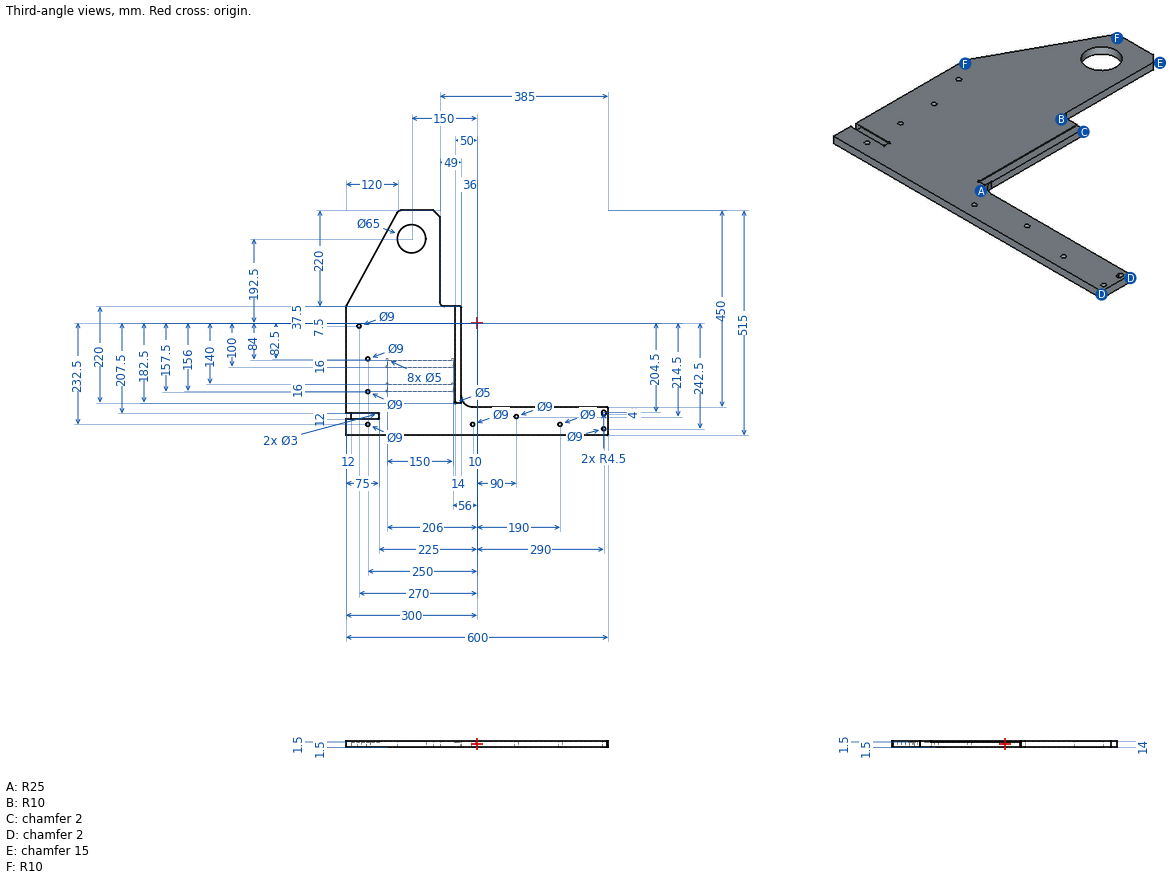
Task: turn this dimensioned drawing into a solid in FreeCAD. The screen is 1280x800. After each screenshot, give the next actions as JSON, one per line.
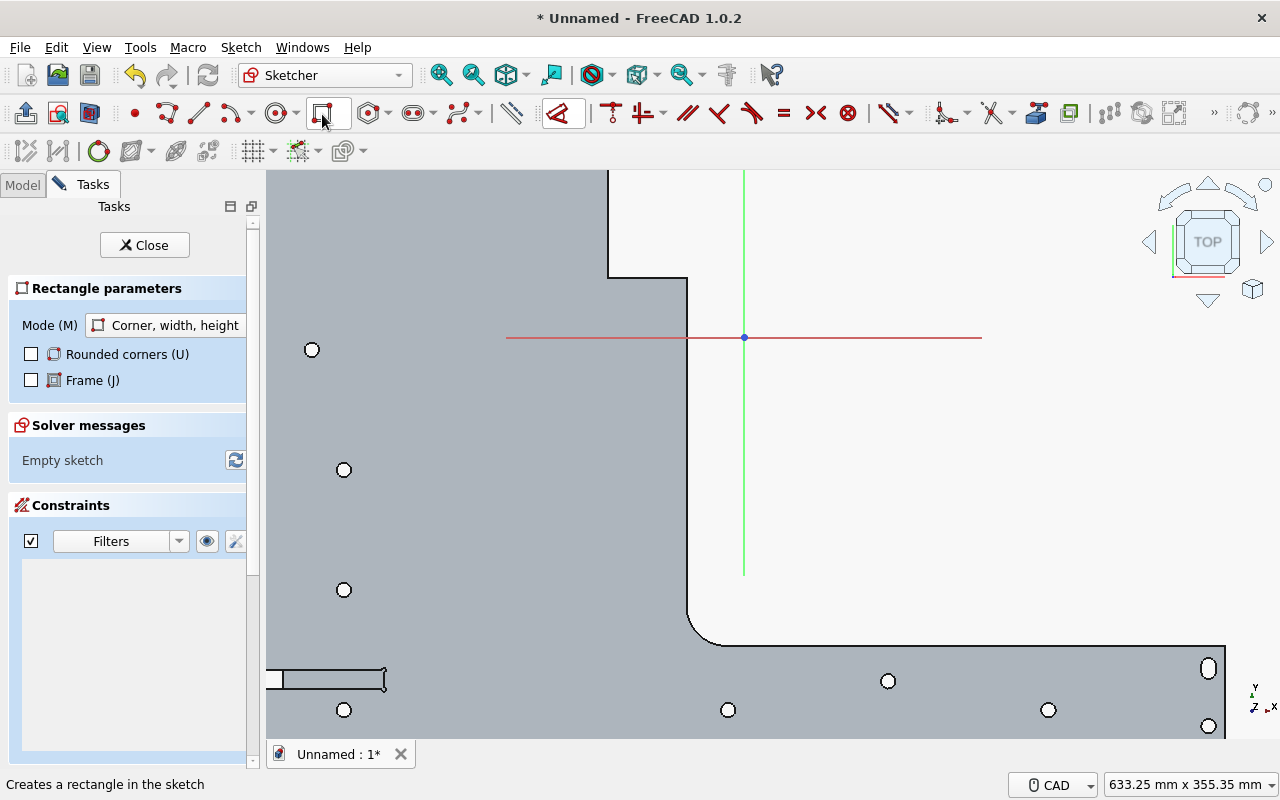
{"action": "left_click", "coordinate": [664, 278]}
{"action": "mouse_move", "coordinate": [687, 630]}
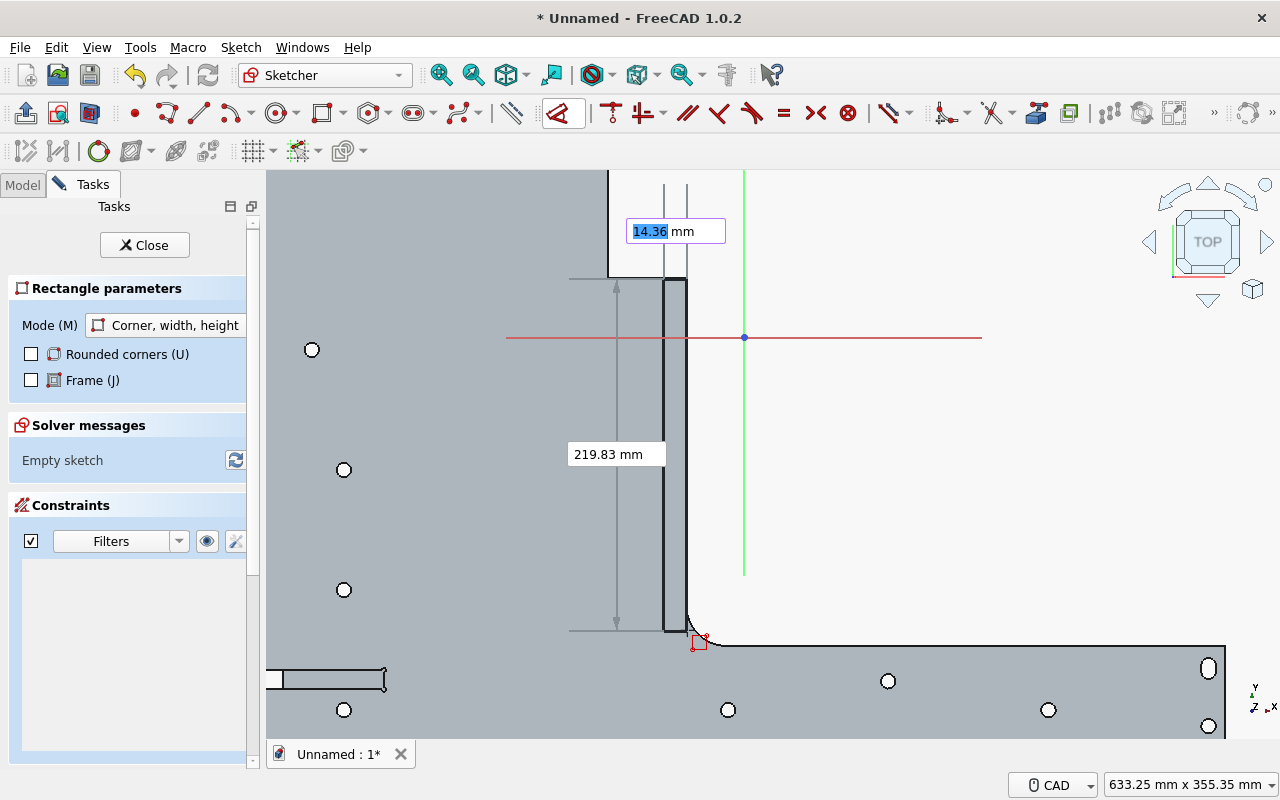
{"action": "type", "text": "14"}
{"action": "key", "text": "Tab"}
{"action": "type", "text": "220"}
{"action": "key", "text": "Return"}
{"action": "key", "text": "Escape"}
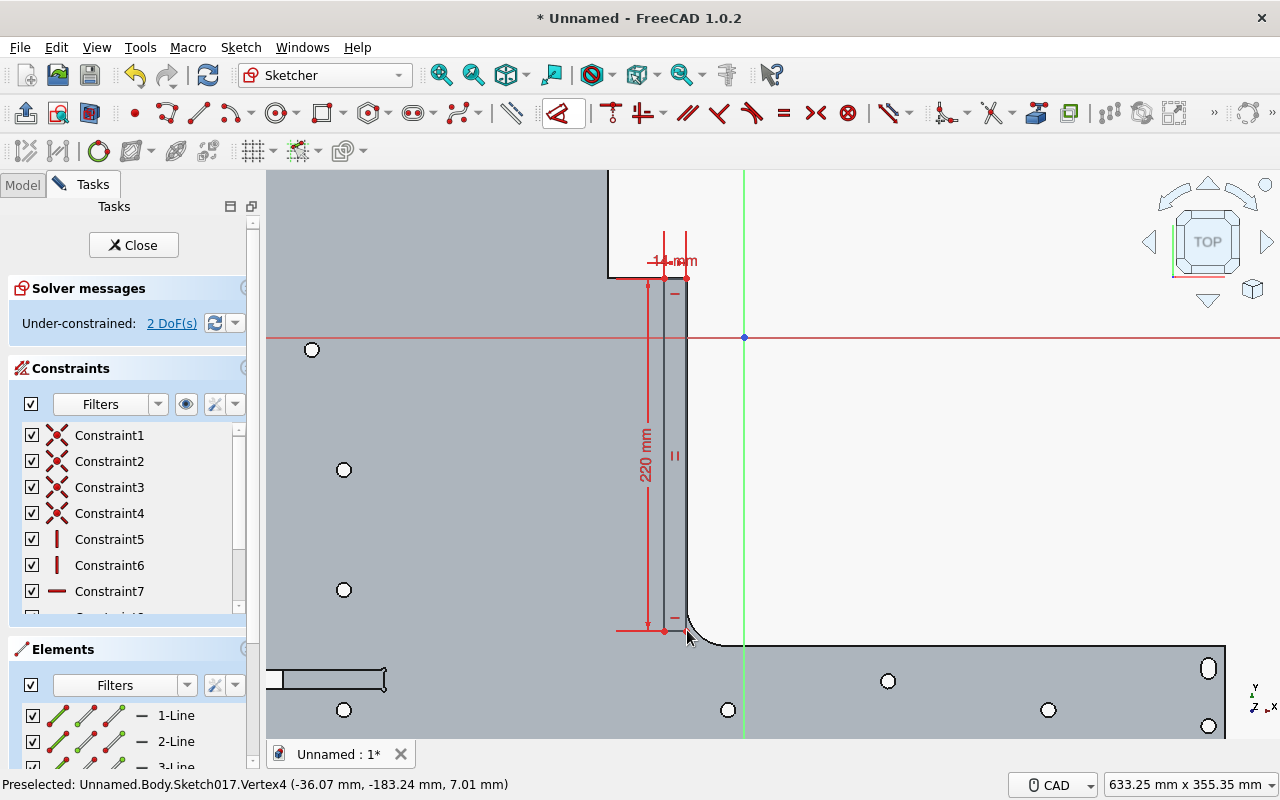
{"action": "left_click", "coordinate": [664, 279]}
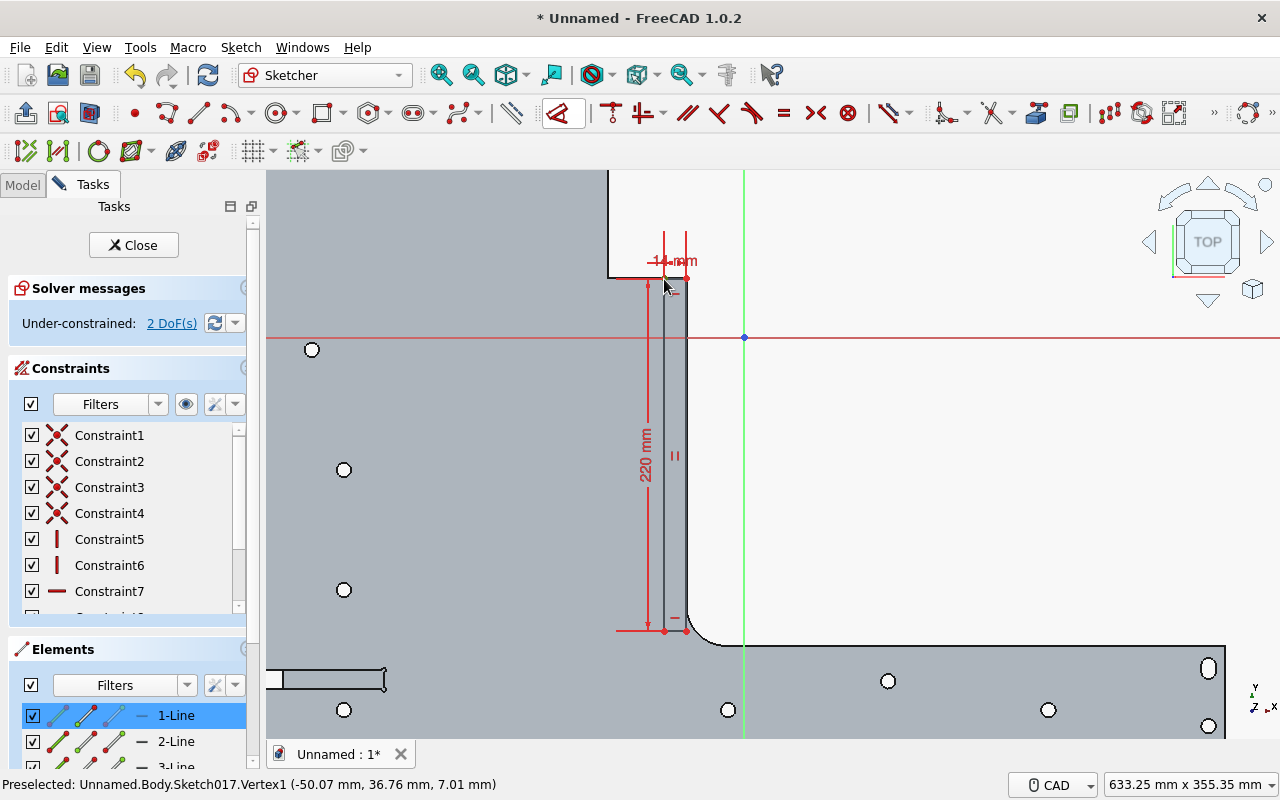
{"action": "key", "text": "l"}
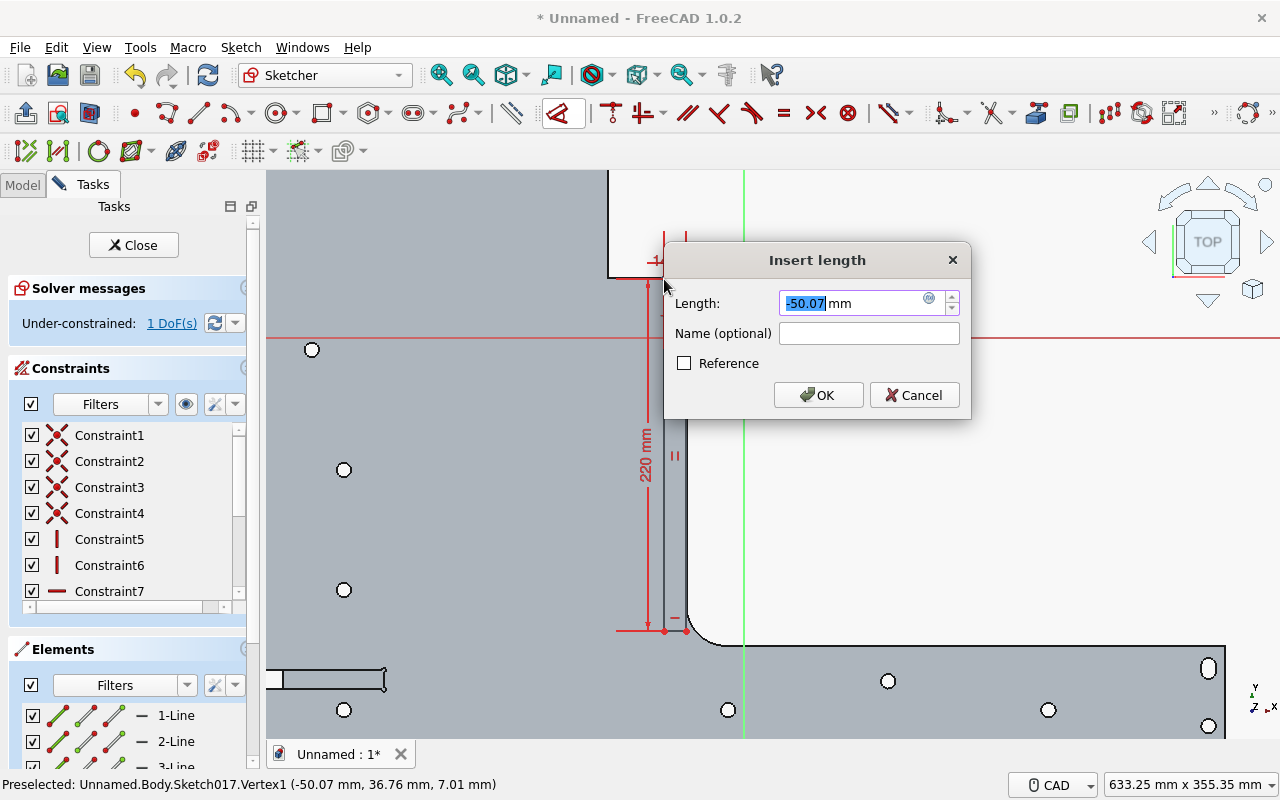
{"action": "type", "text": "-50"}
{"action": "key", "text": "Return"}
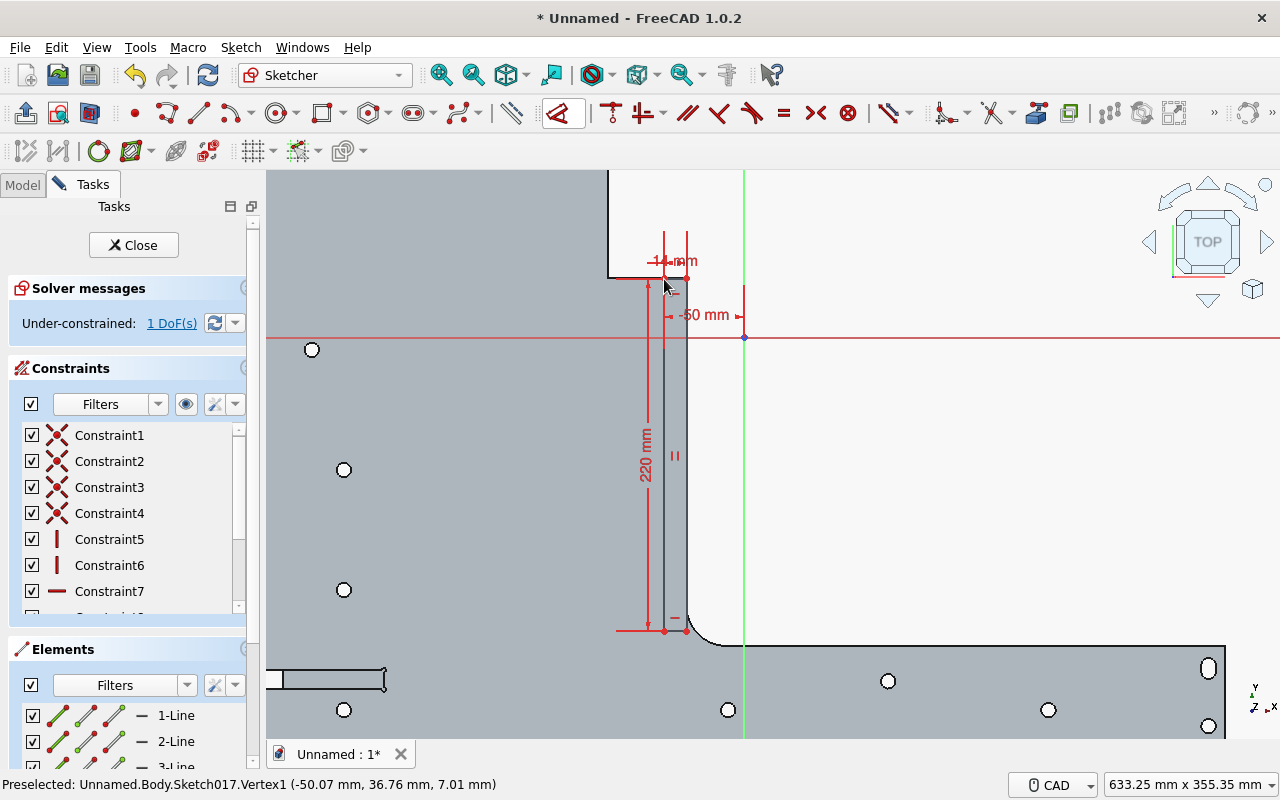
{"action": "left_click", "coordinate": [664, 279]}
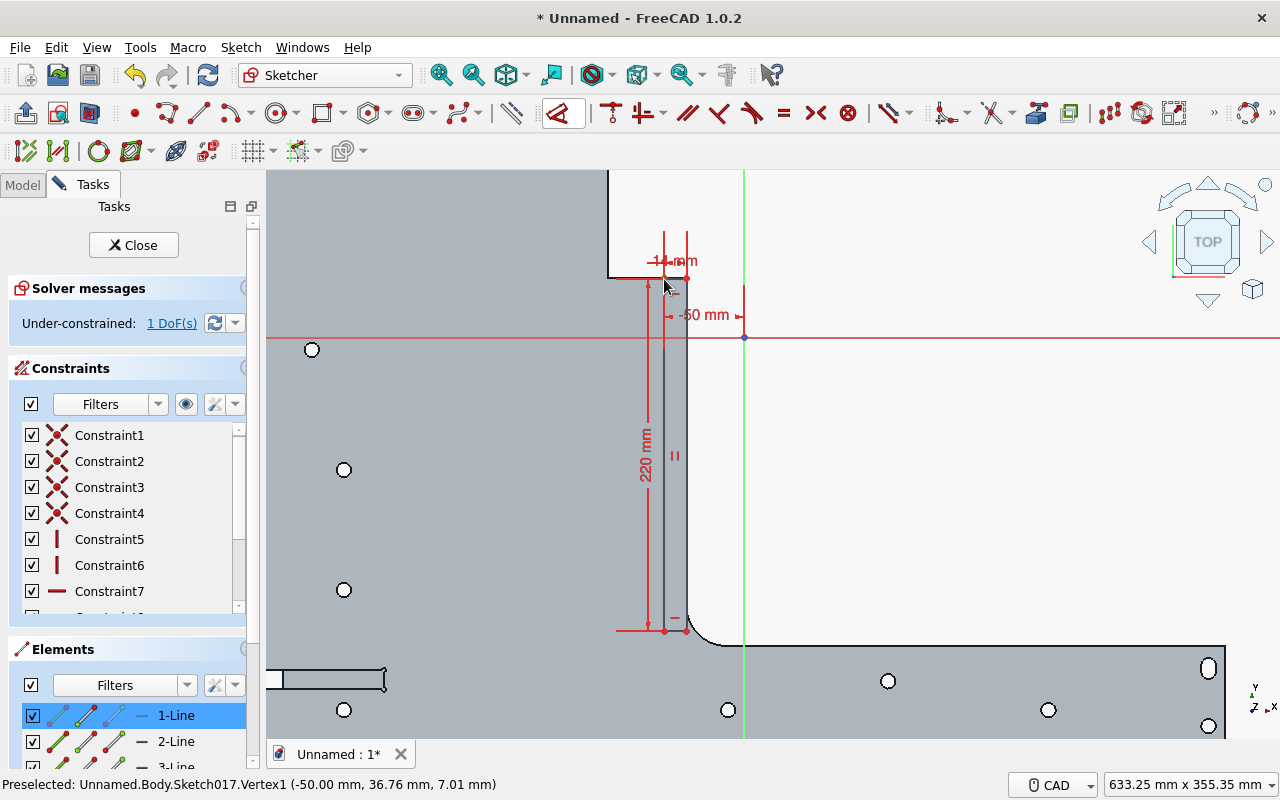
{"action": "key", "text": "i"}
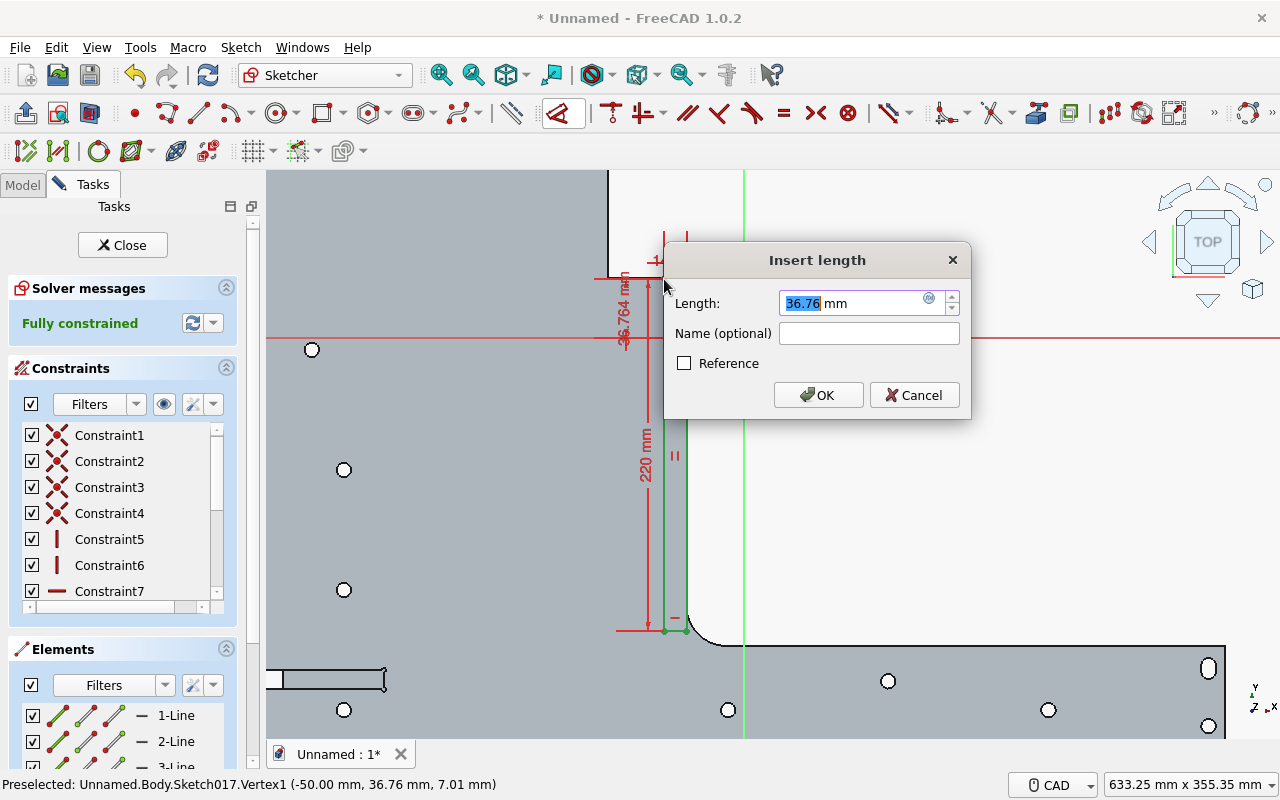
{"action": "type", "text": "37.5"}
{"action": "key", "text": "Return"}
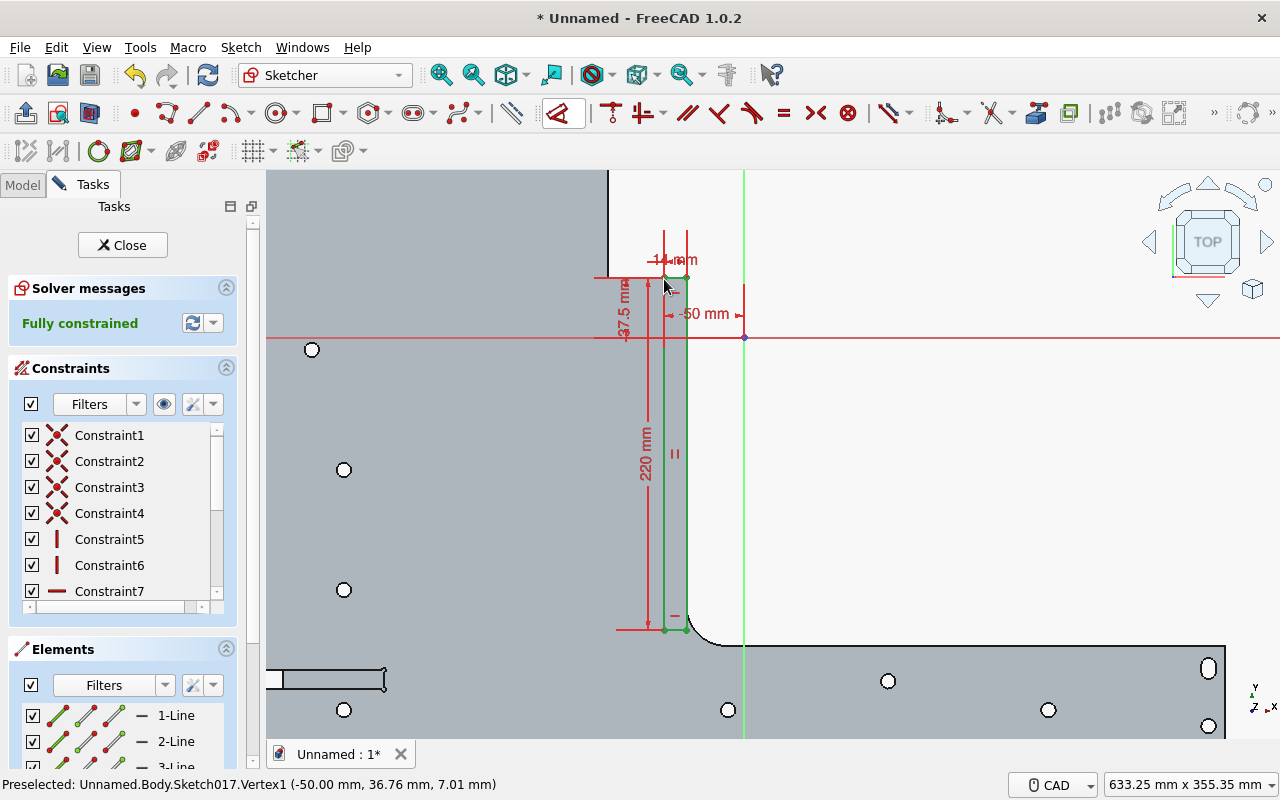
{"action": "left_click", "coordinate": [123, 245]}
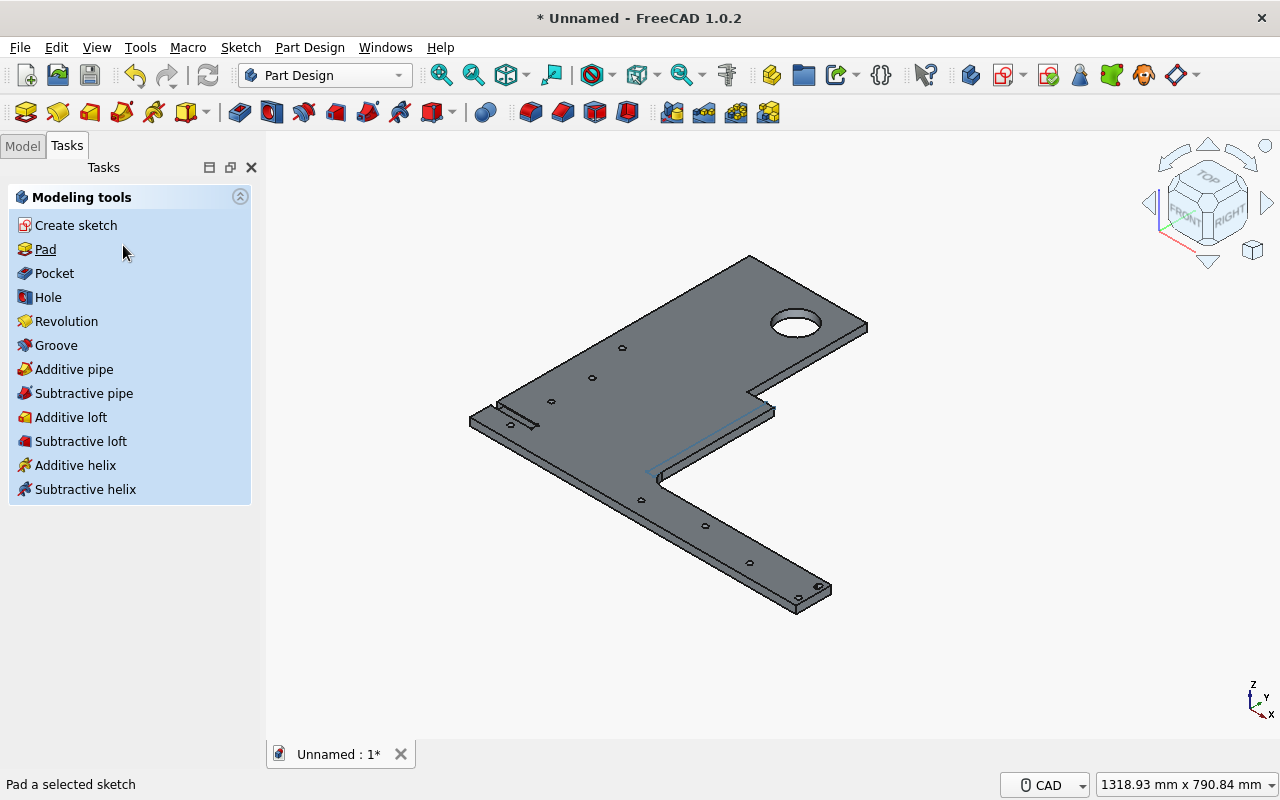
{"action": "left_click", "coordinate": [240, 112]}